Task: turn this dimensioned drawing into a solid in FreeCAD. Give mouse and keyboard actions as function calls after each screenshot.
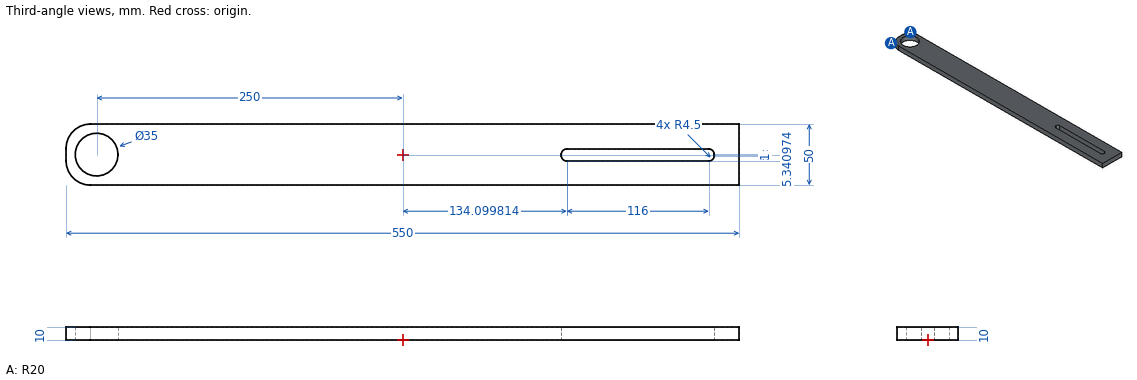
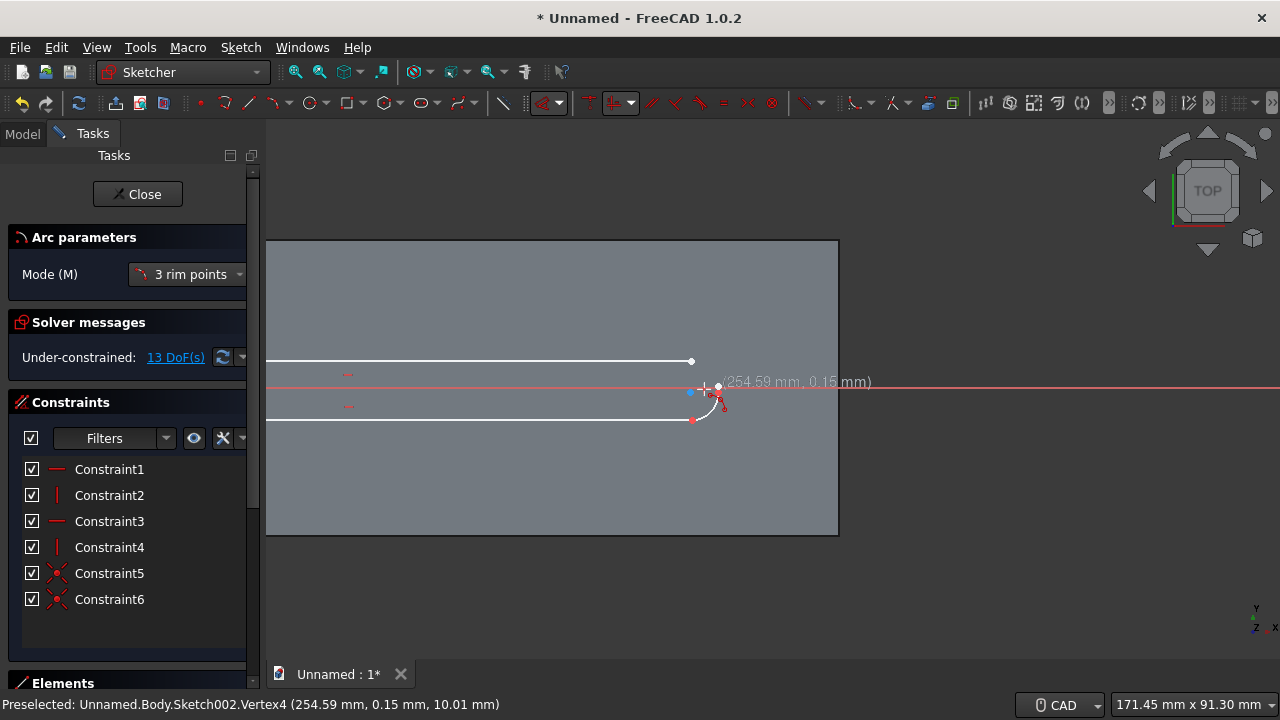
scroll(1115, 389, down, 5)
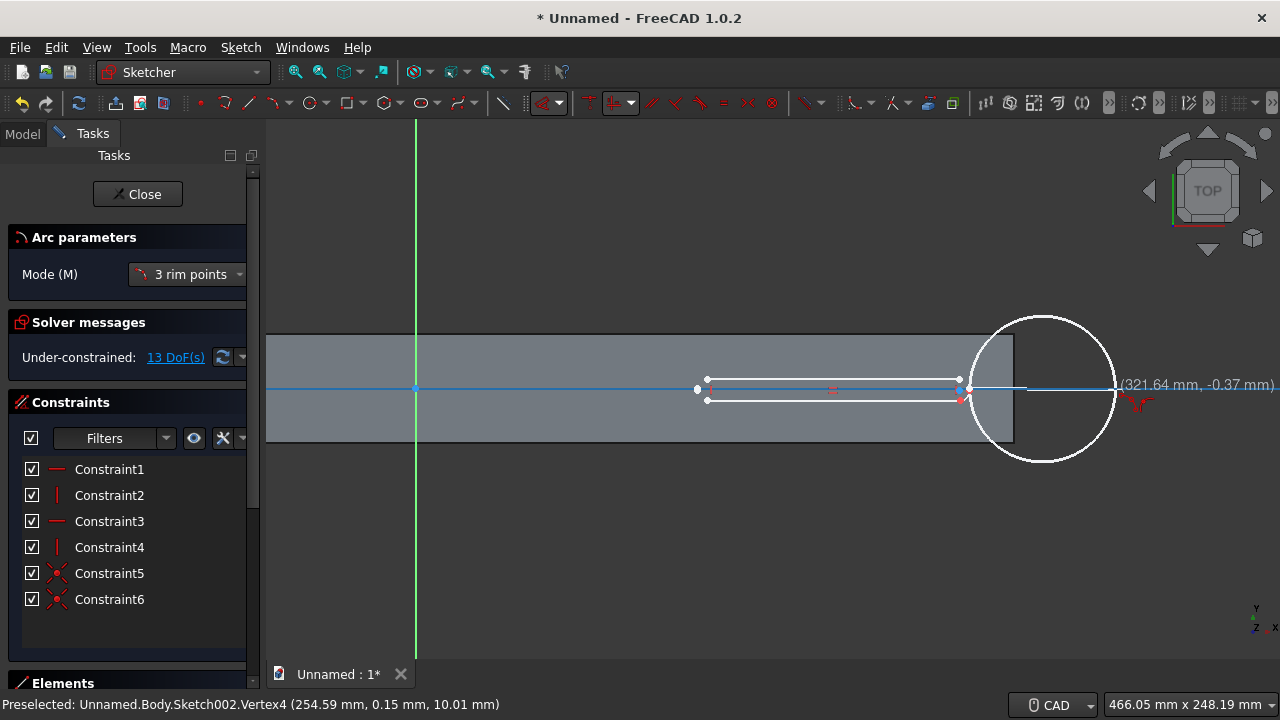
scroll(960, 379, up, 3)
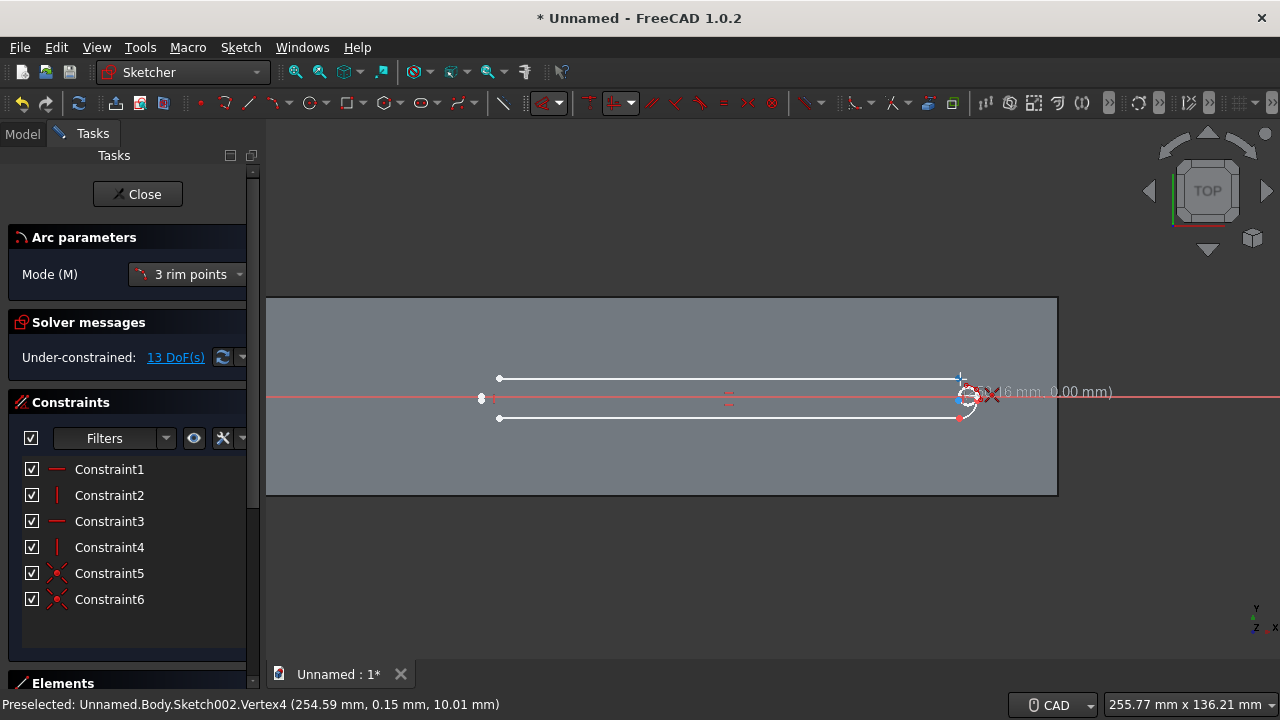
click(959, 379)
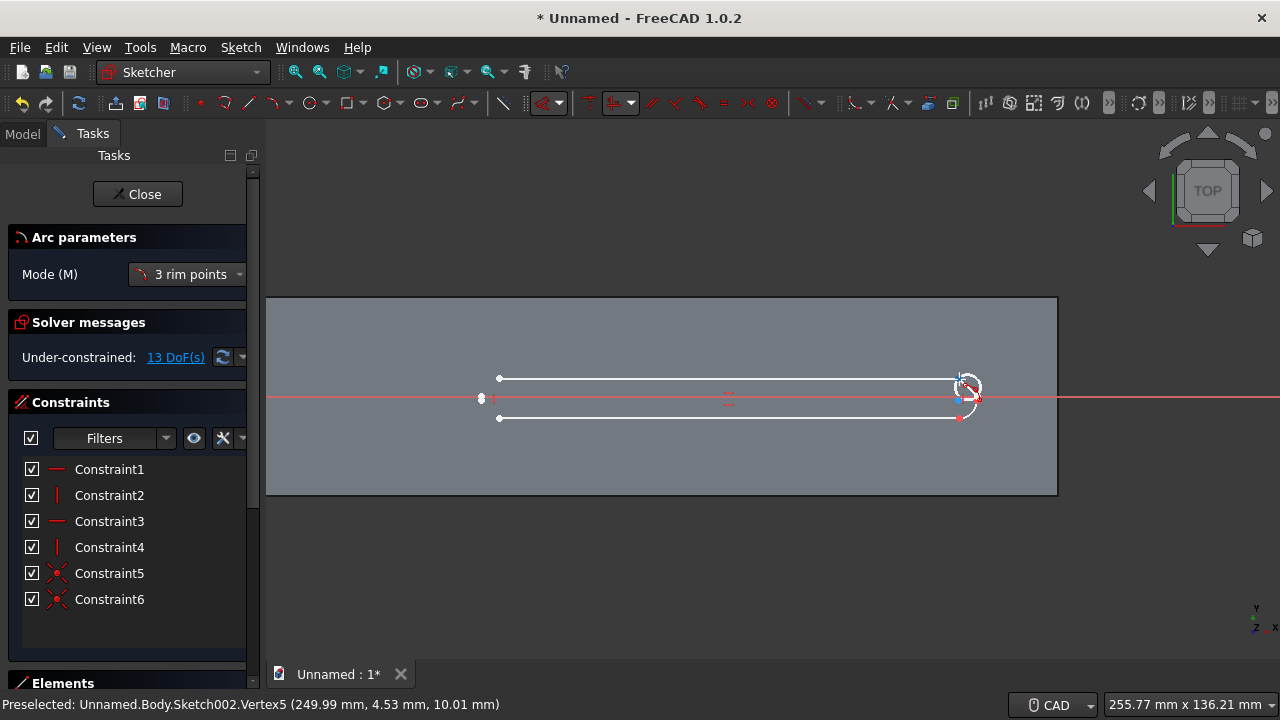
scroll(972, 383, up, 6)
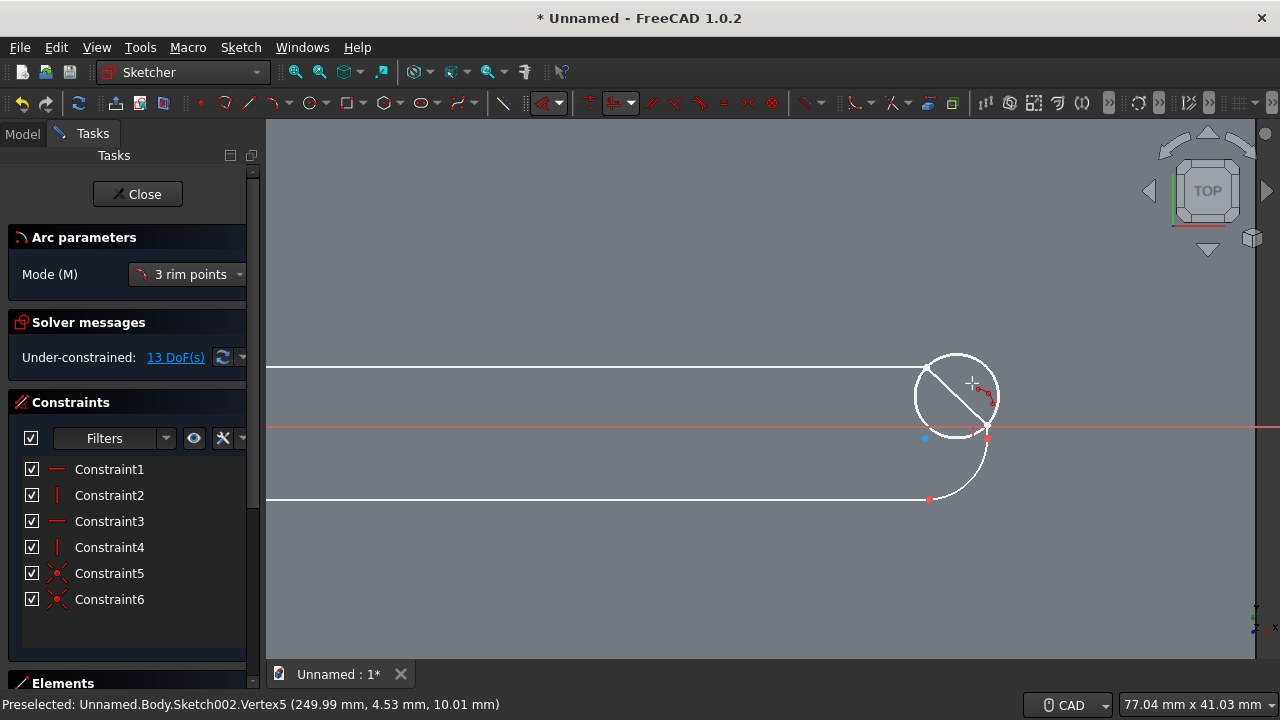
click(970, 383)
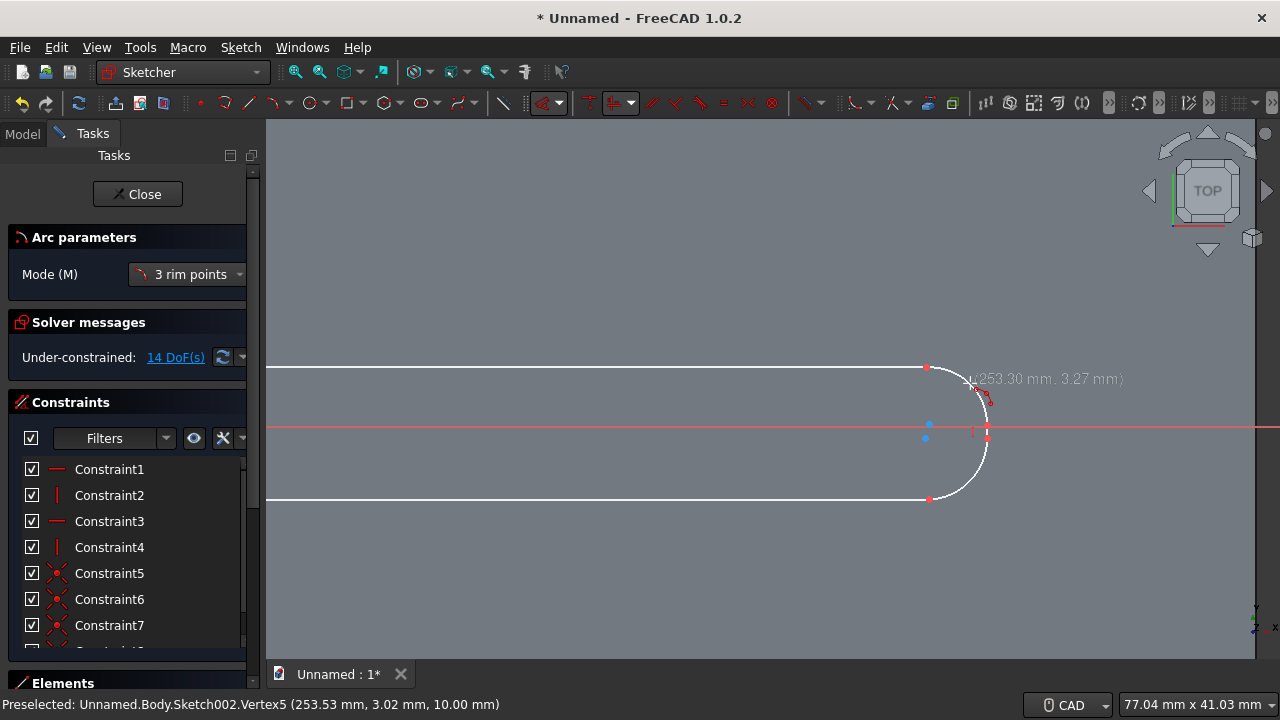
scroll(980, 381, down, 9)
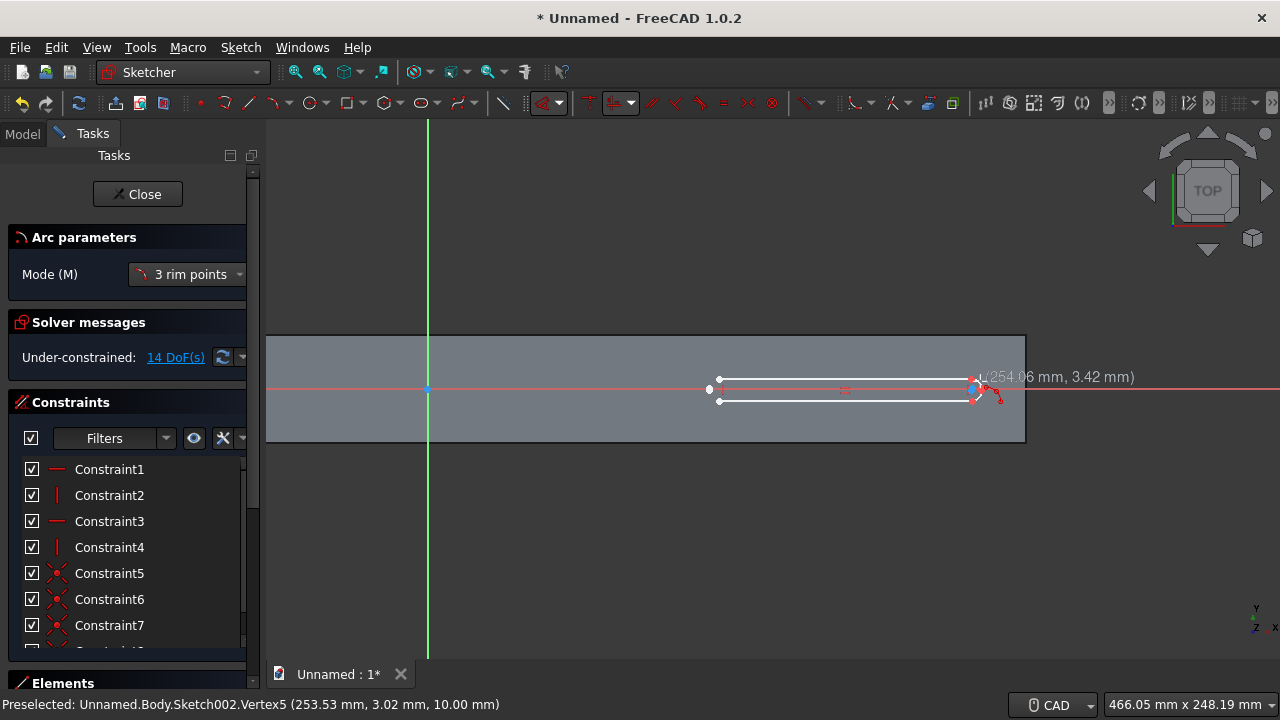
scroll(720, 379, up, 3)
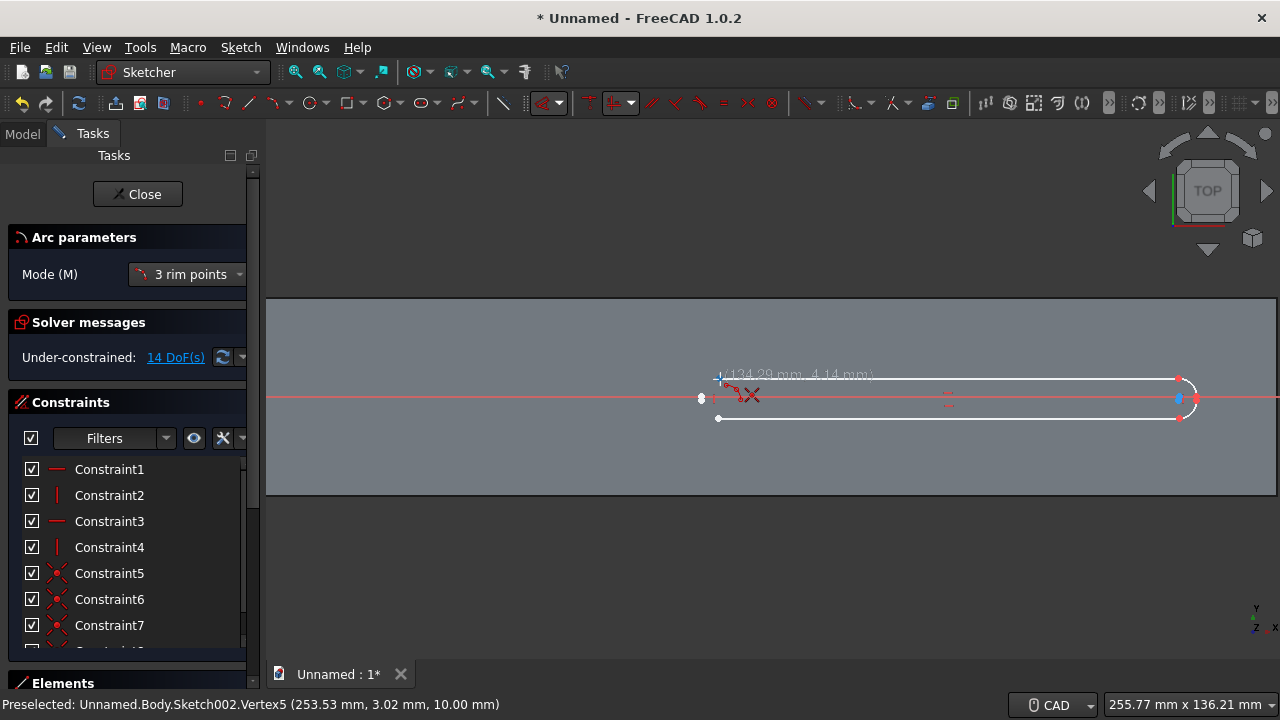
click(719, 379)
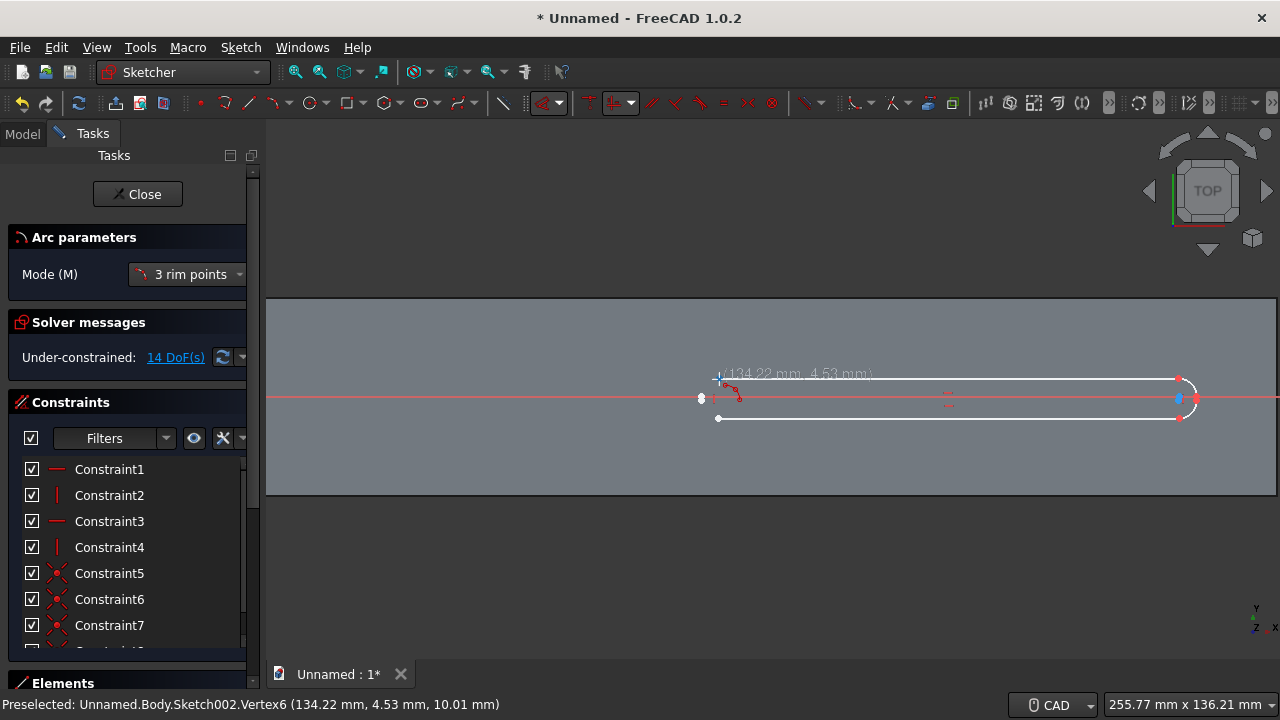
scroll(701, 396, up, 17)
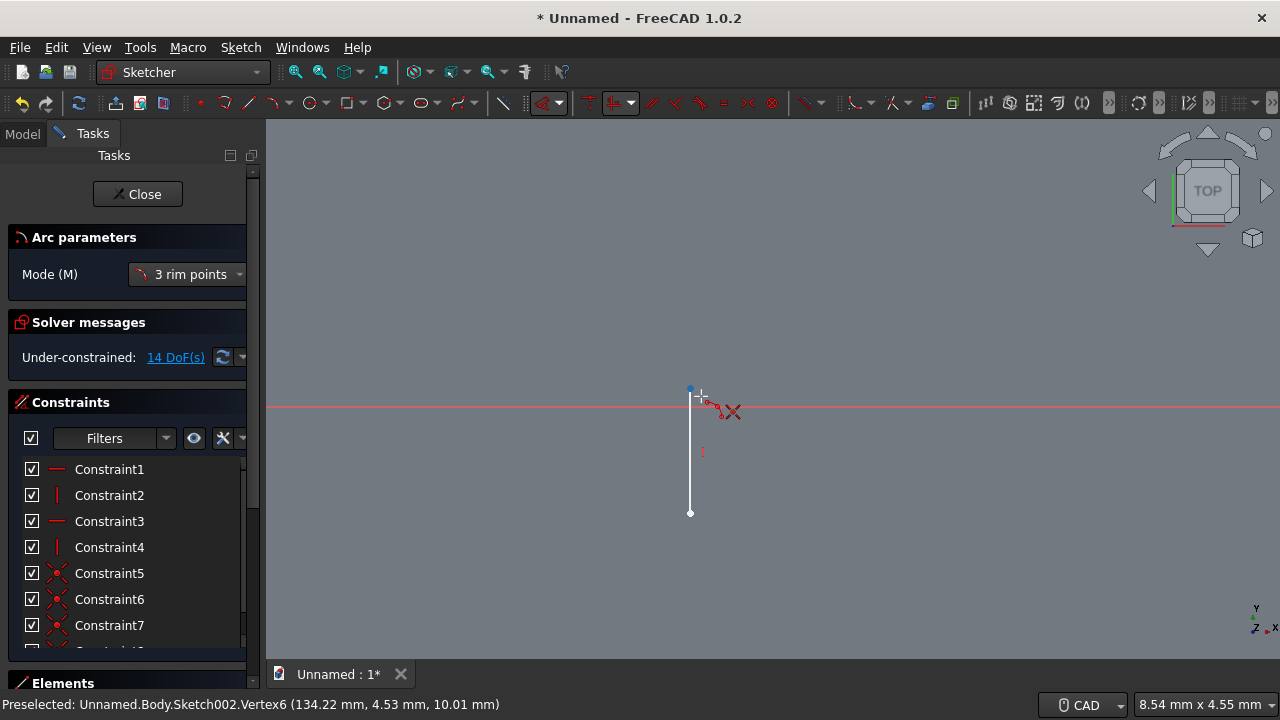
click(690, 389)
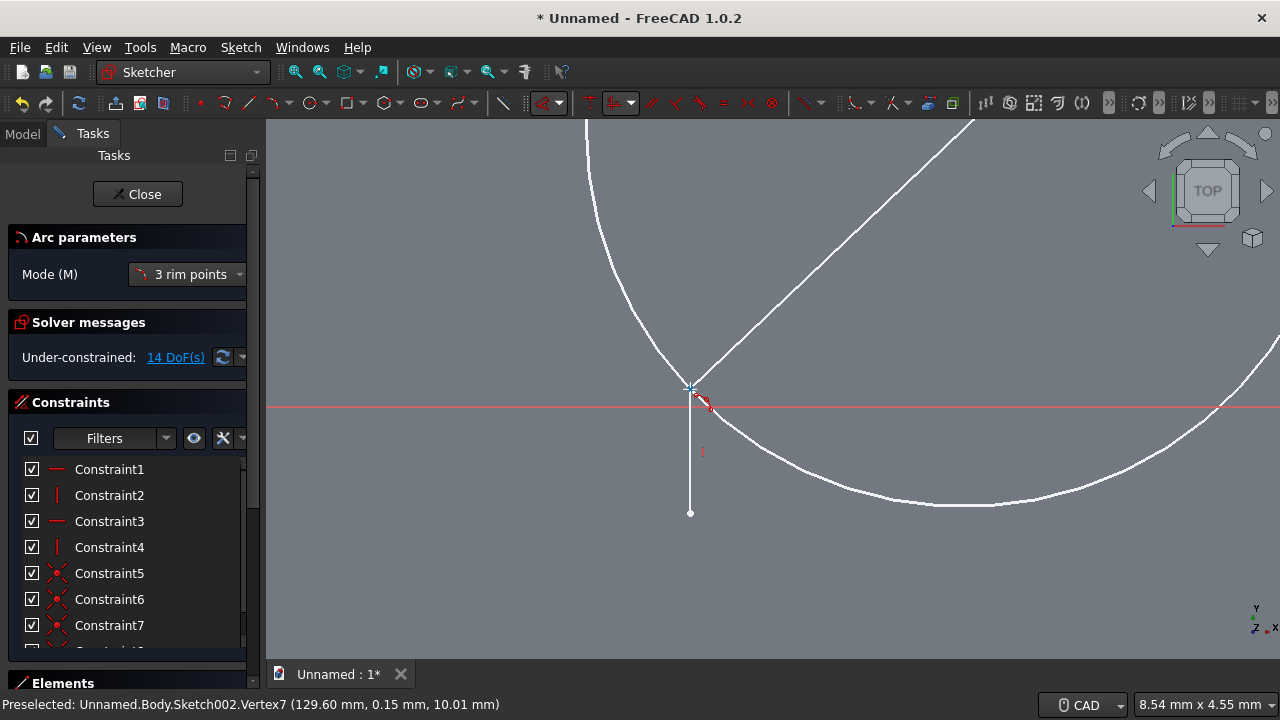
scroll(704, 389, down, 15)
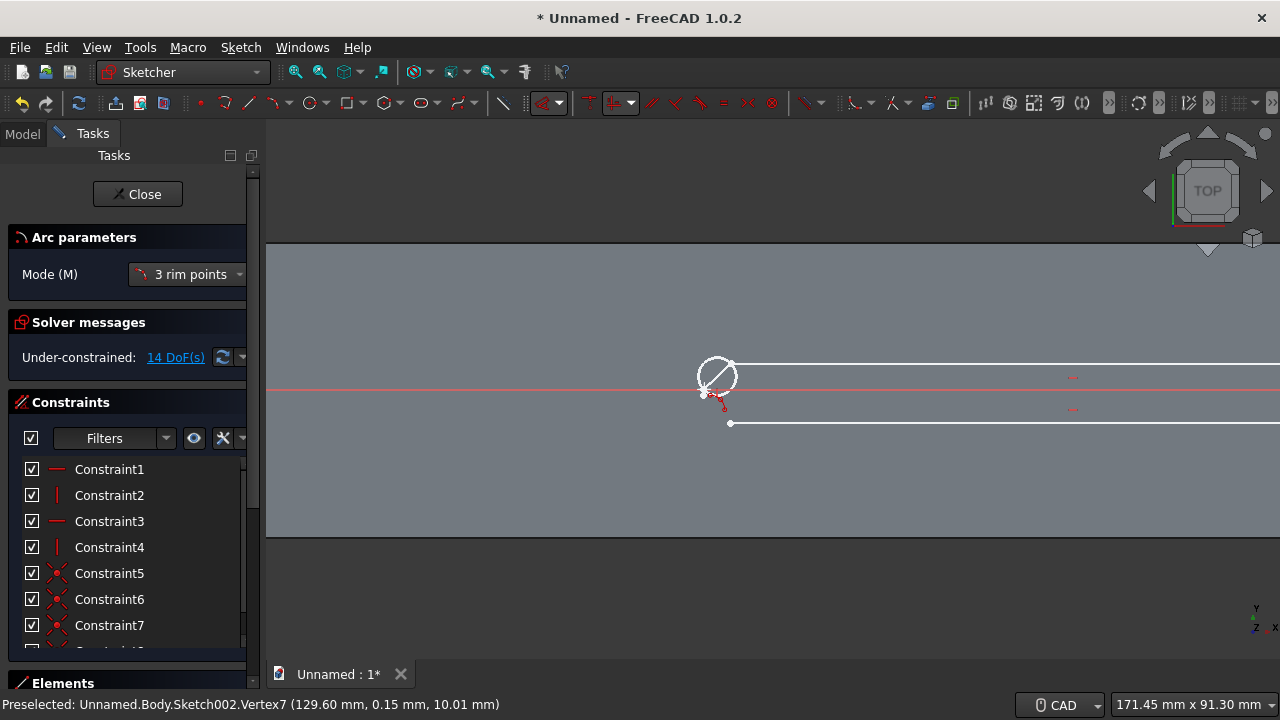
scroll(713, 387, down, 5)